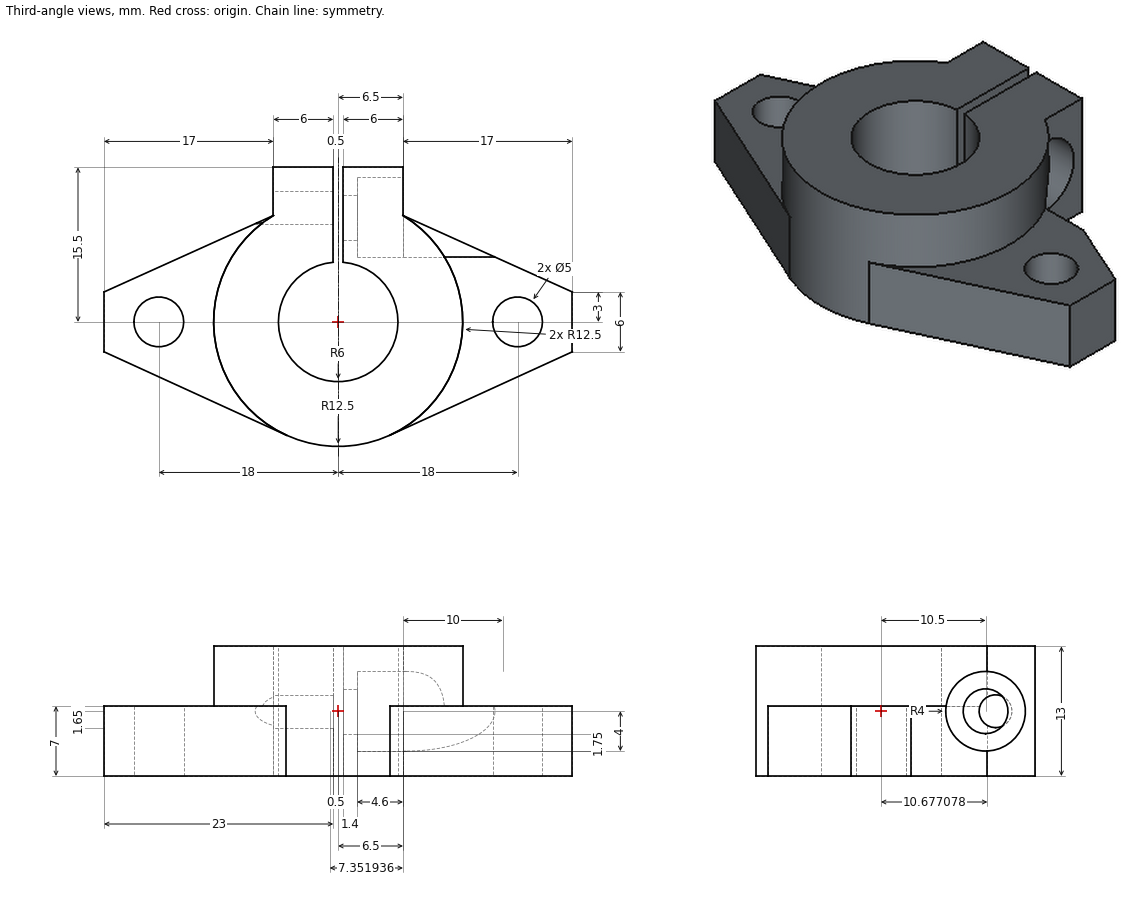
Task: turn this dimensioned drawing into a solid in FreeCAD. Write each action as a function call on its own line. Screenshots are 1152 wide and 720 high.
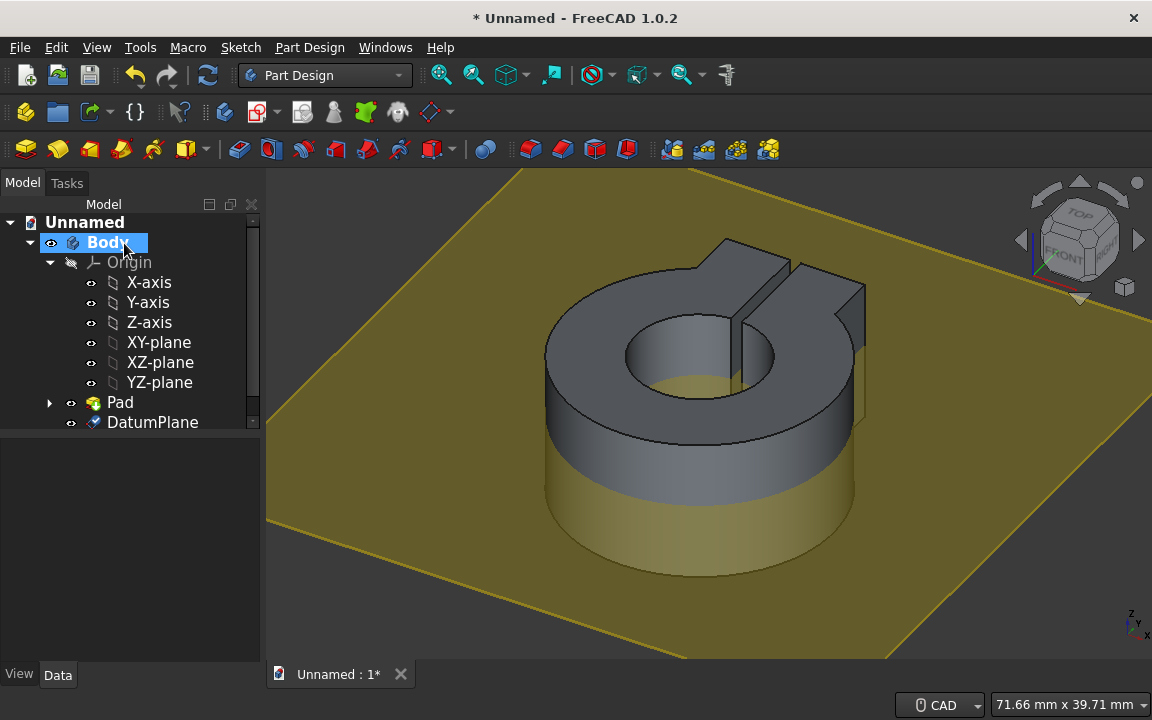
click(116, 423)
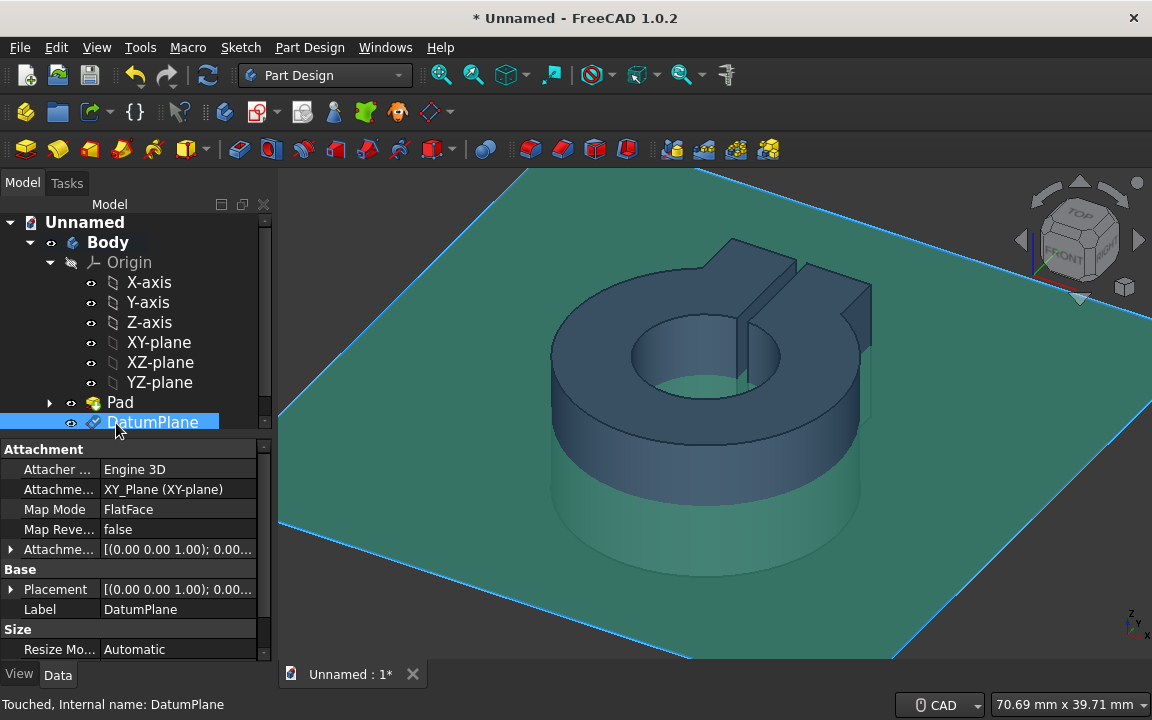
click(258, 112)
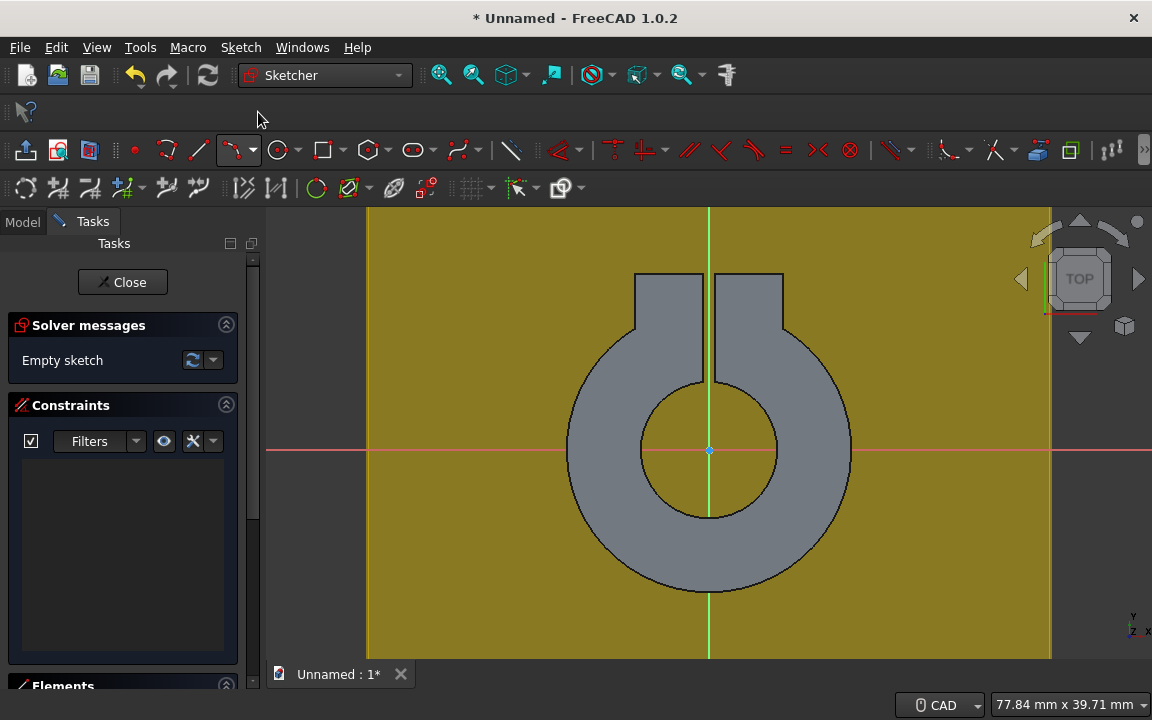
click(90, 150)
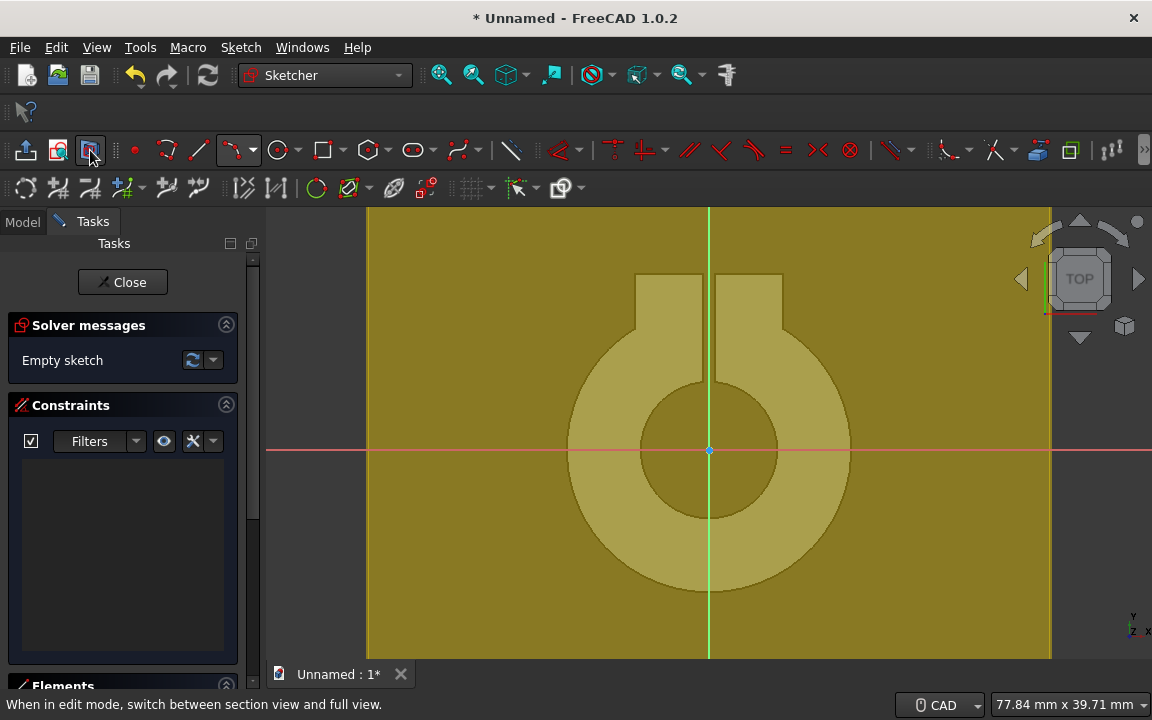
scroll(331, 338, down, 1)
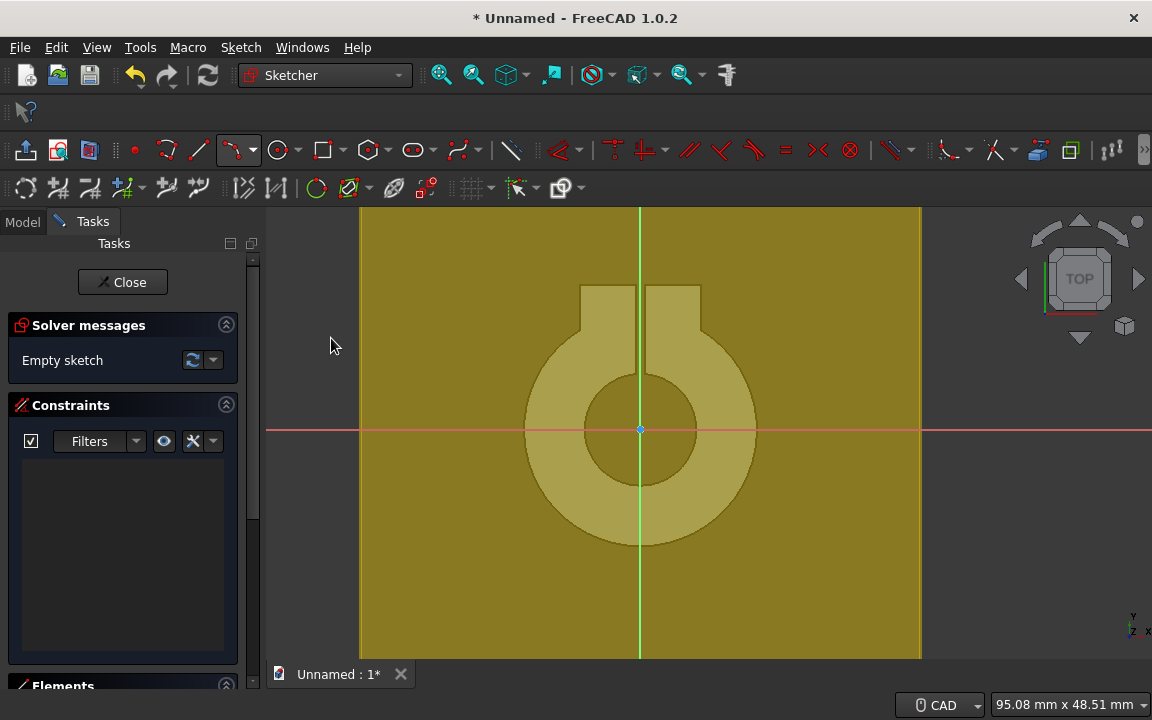
click(168, 150)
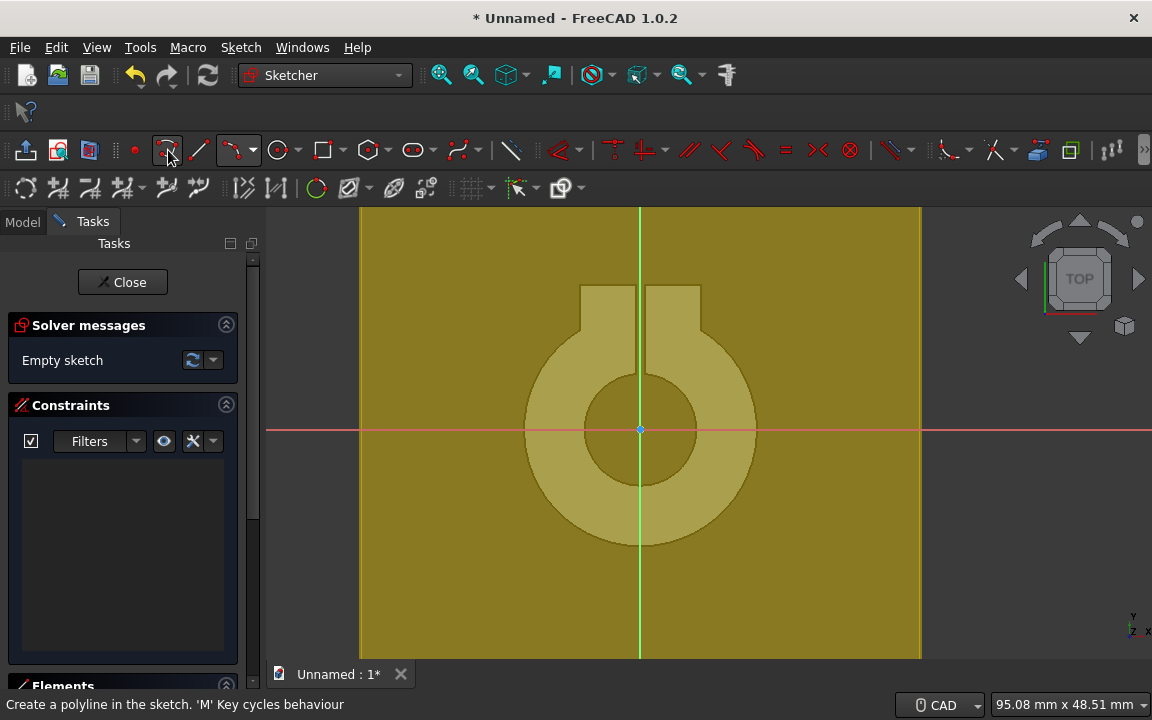
click(701, 330)
click(859, 402)
click(859, 458)
click(689, 536)
right_click(689, 536)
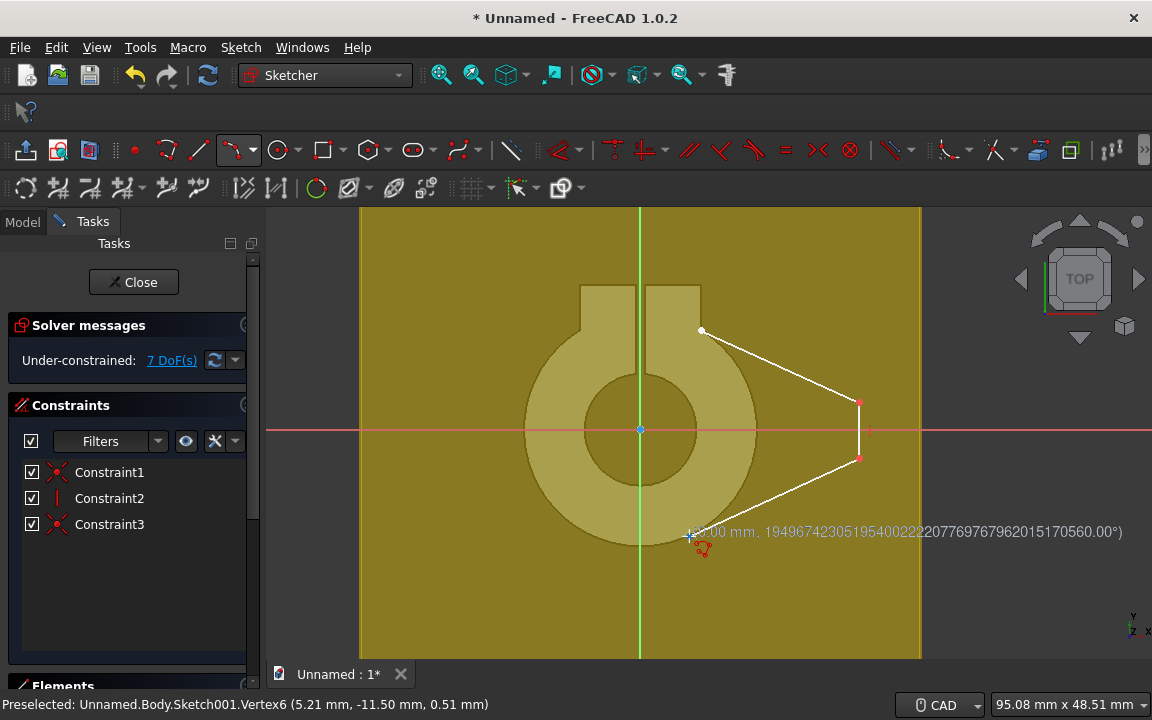
click(232, 150)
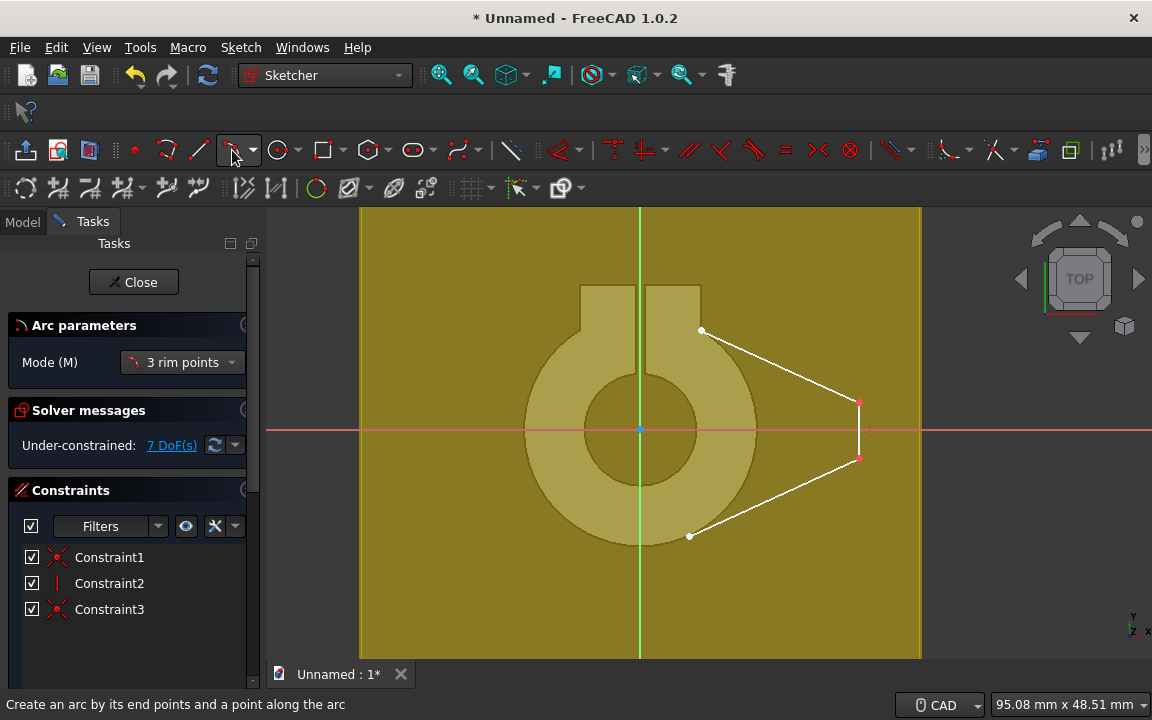
click(689, 537)
click(701, 331)
click(753, 462)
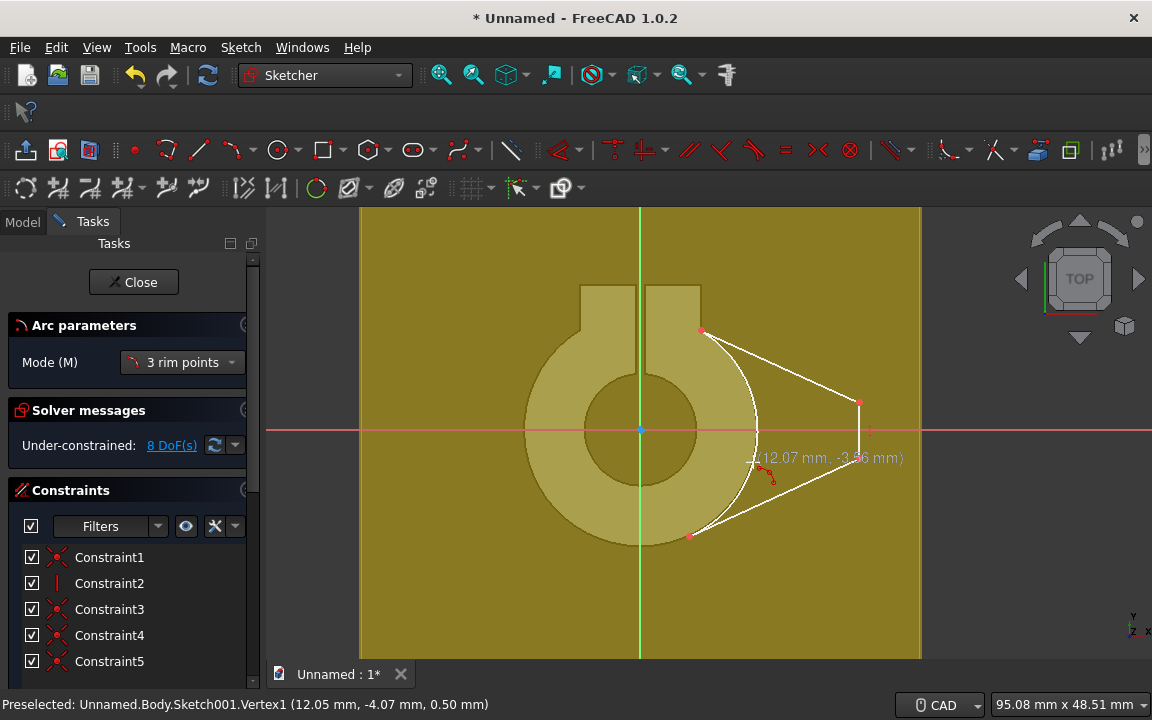
click(168, 150)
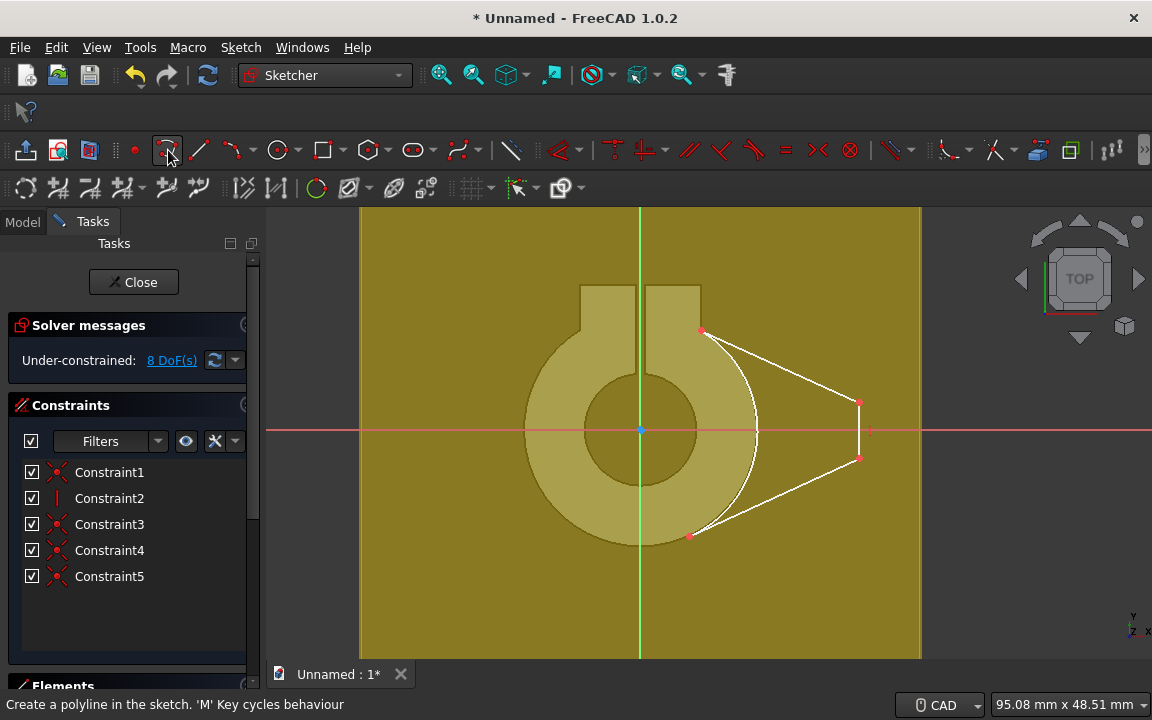
click(592, 536)
click(422, 458)
click(422, 402)
click(580, 330)
right_click(580, 330)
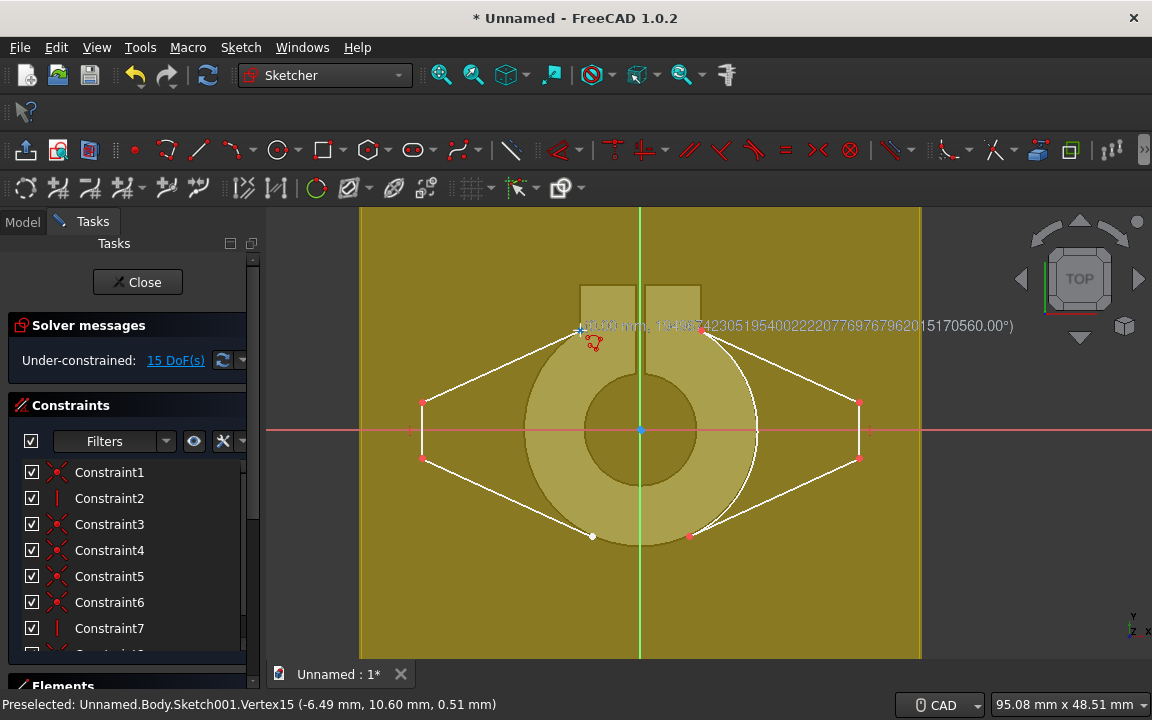
click(232, 150)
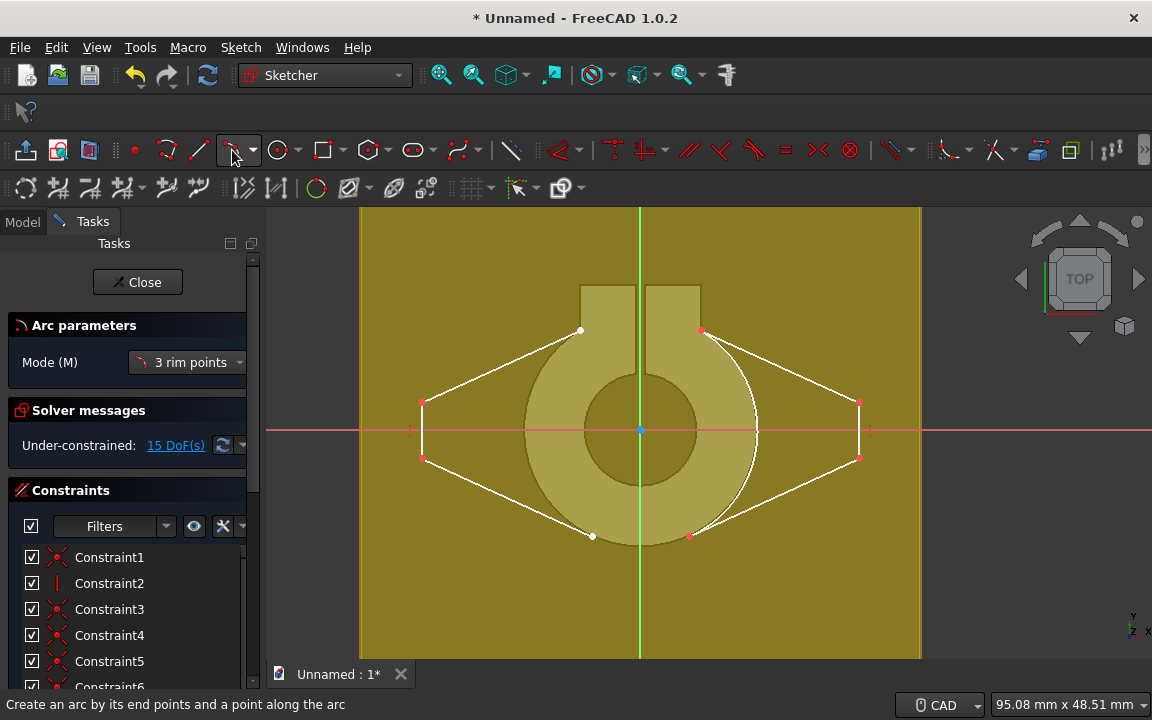
click(580, 331)
click(592, 537)
click(525, 412)